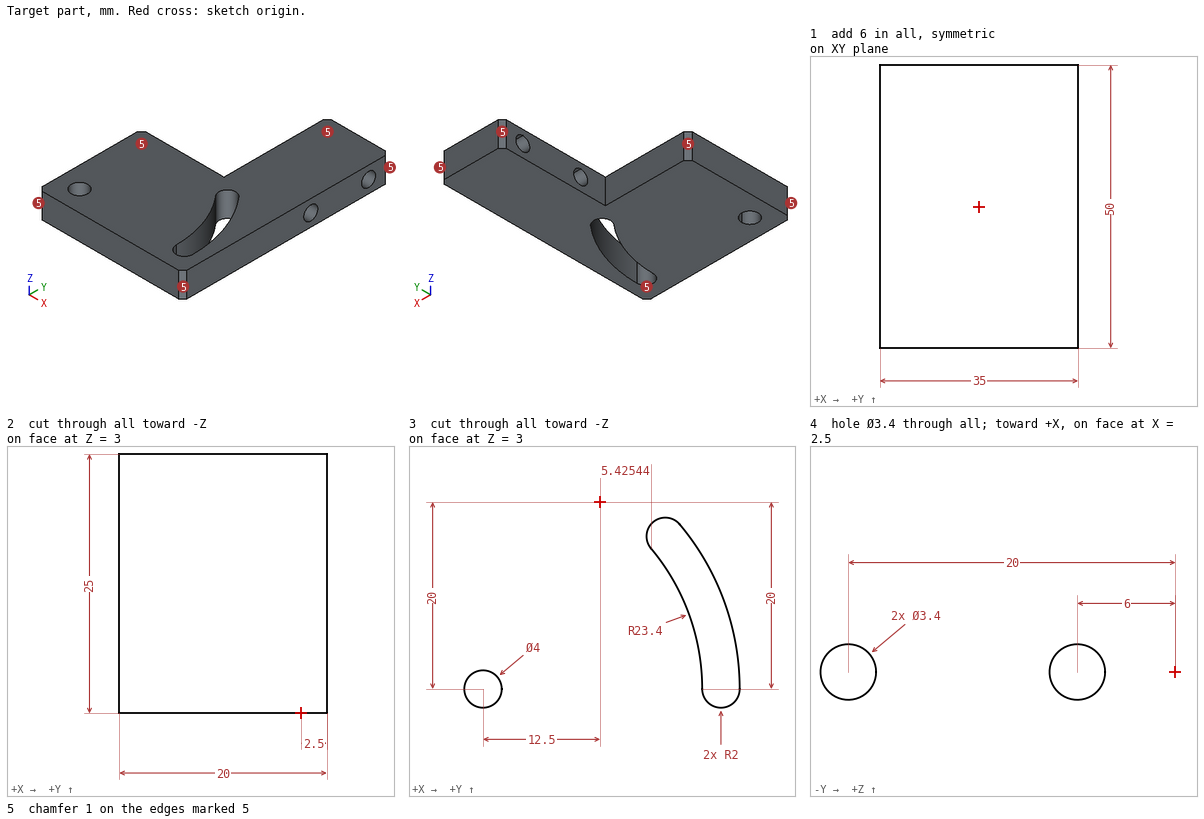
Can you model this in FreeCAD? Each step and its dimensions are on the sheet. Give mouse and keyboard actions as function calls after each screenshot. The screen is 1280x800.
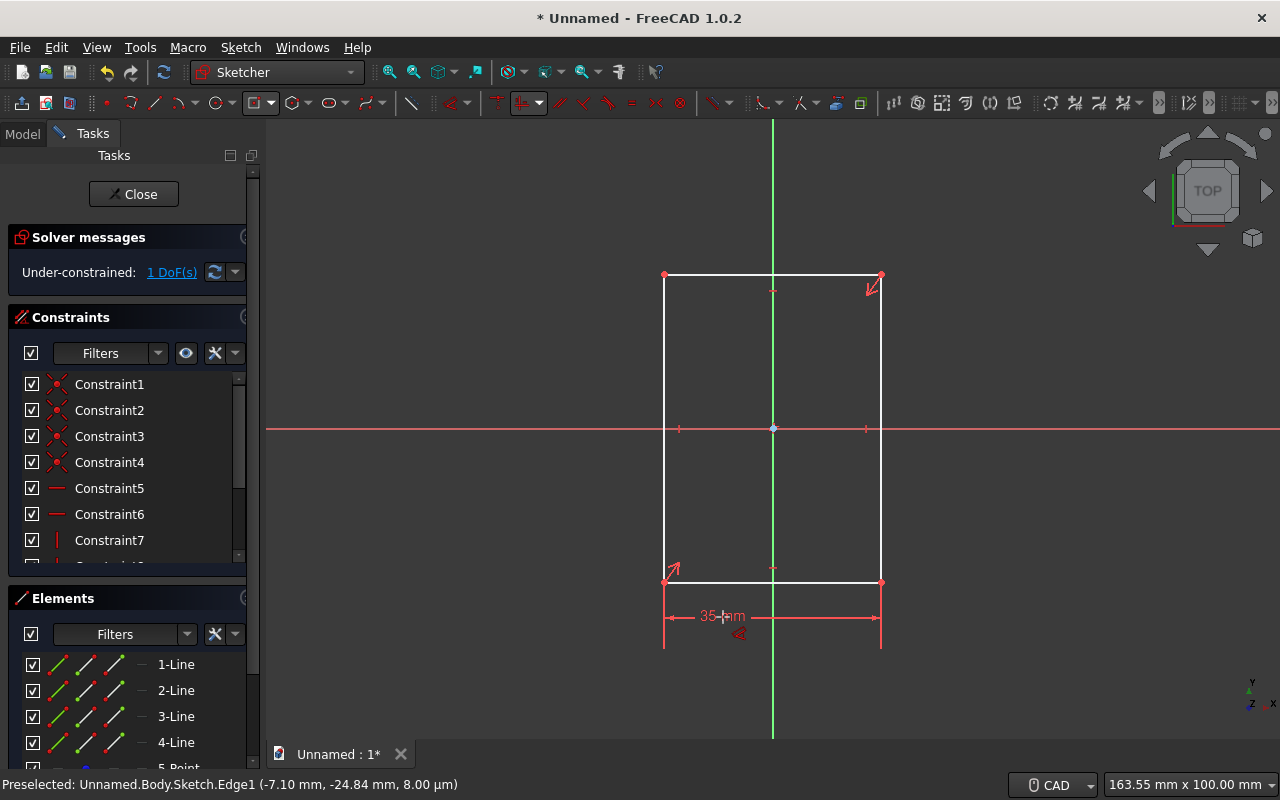
click(882, 491)
click(916, 358)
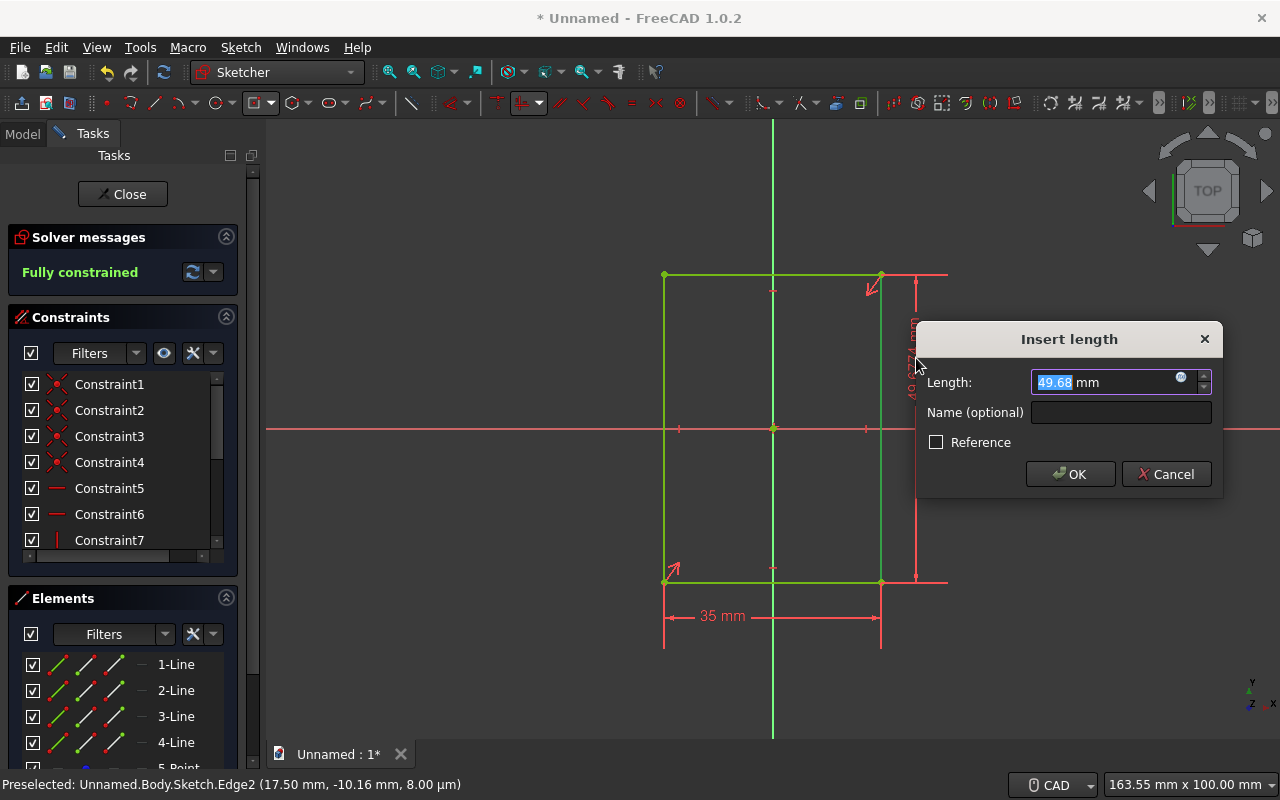
text(50)
key(Return)
key(Escape)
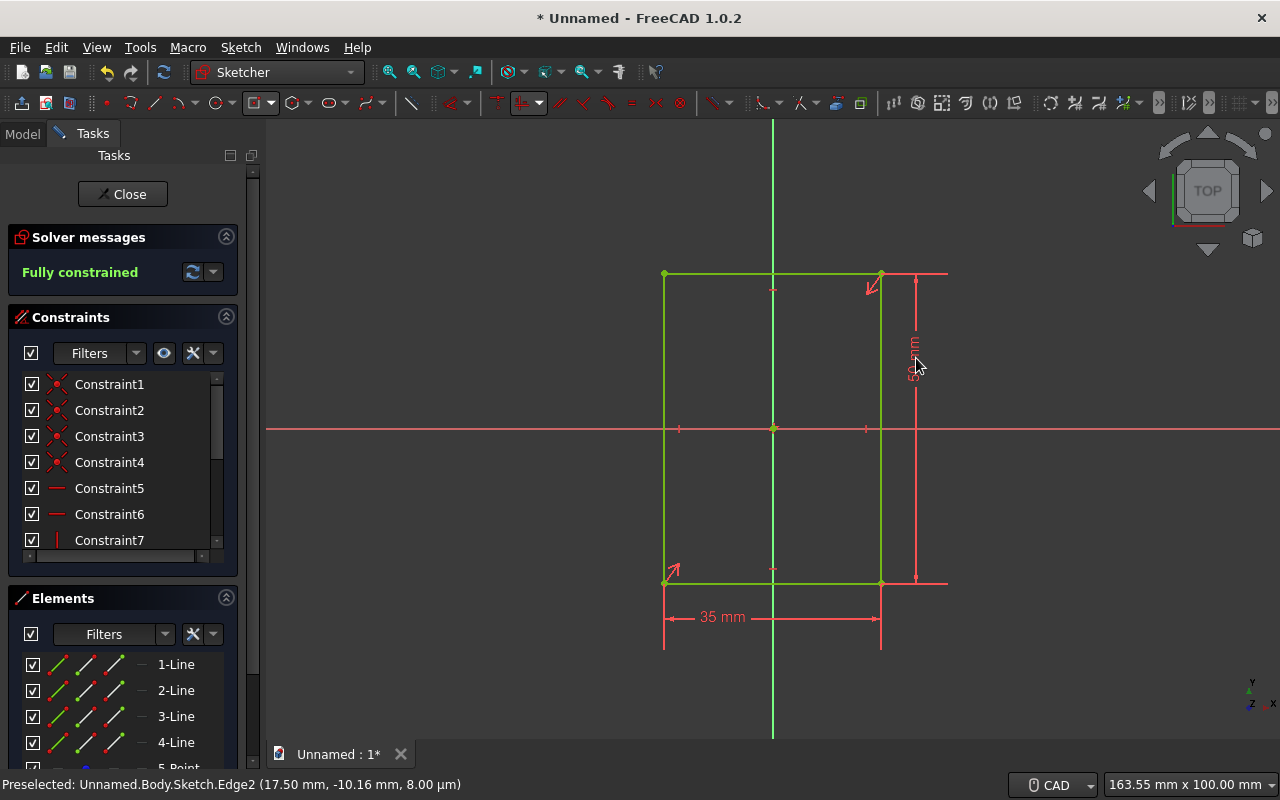
click(123, 194)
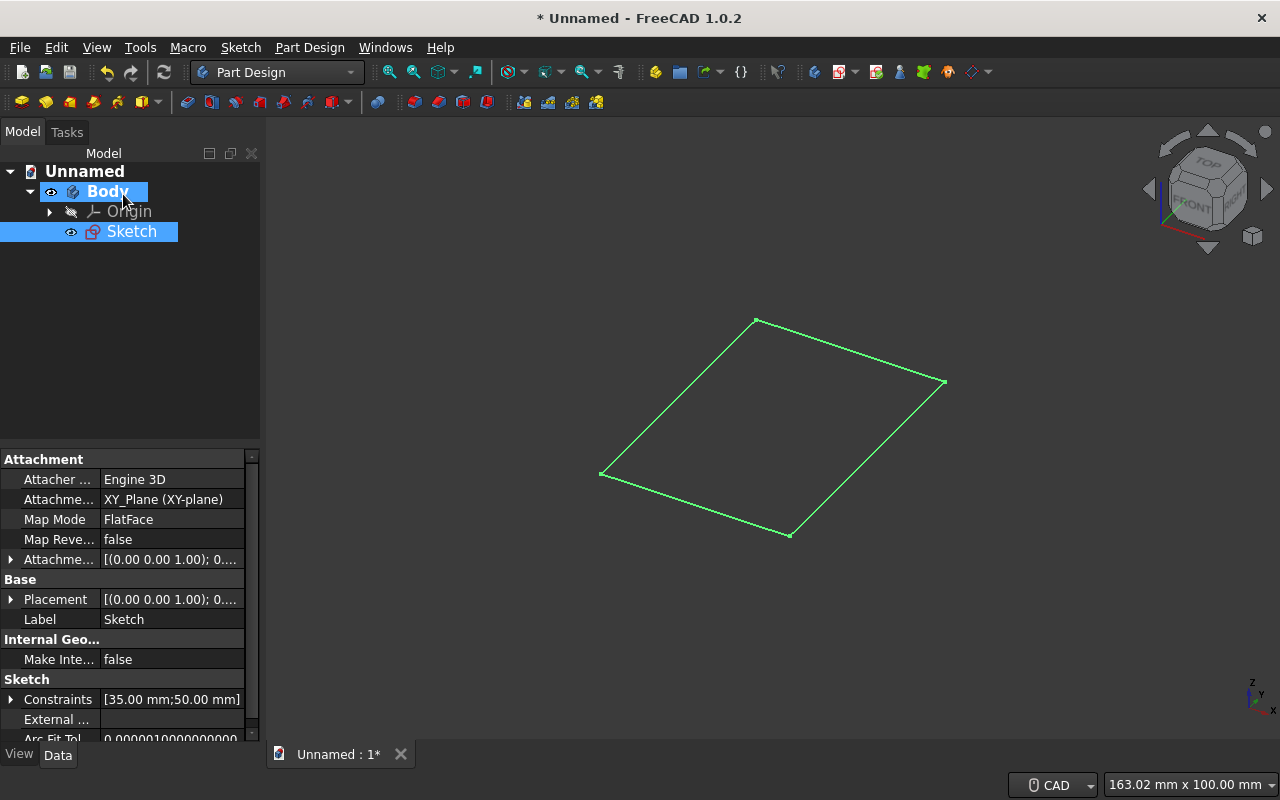
click(22, 102)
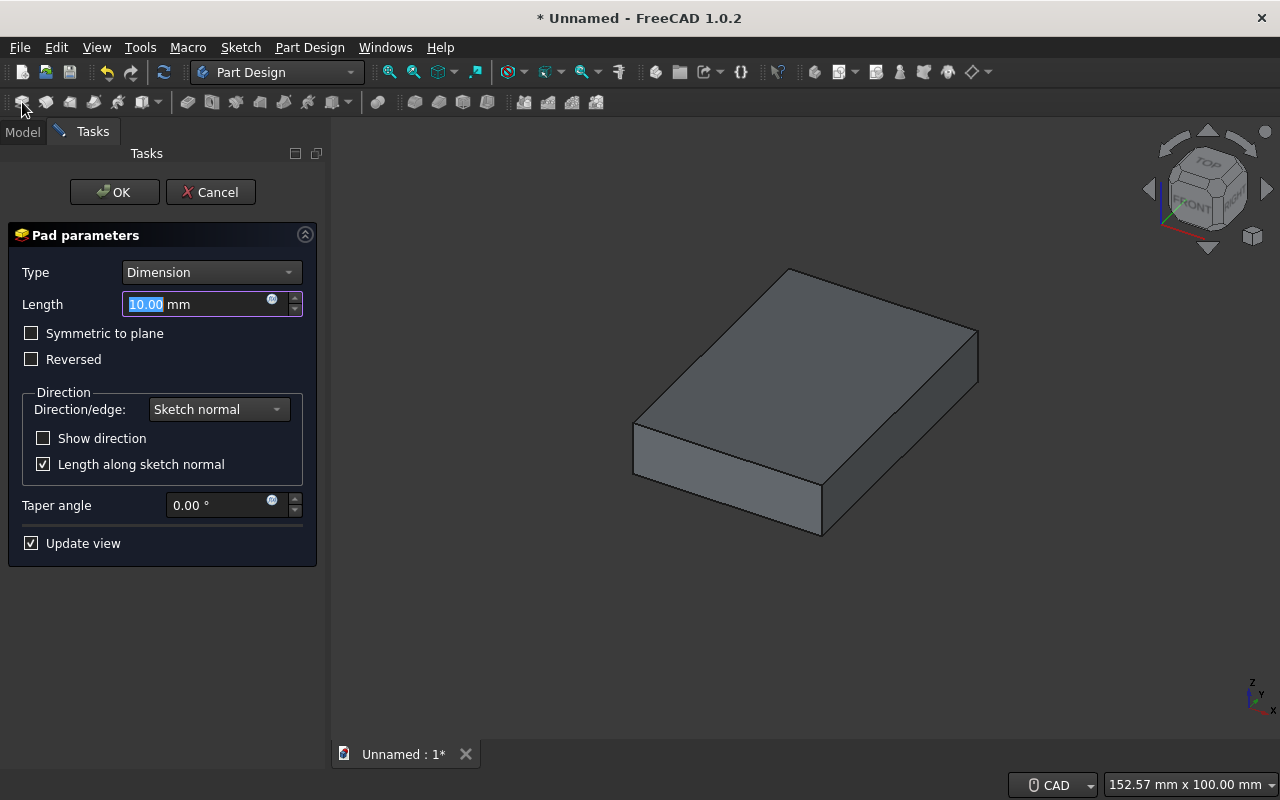
text(6)
key(Tab)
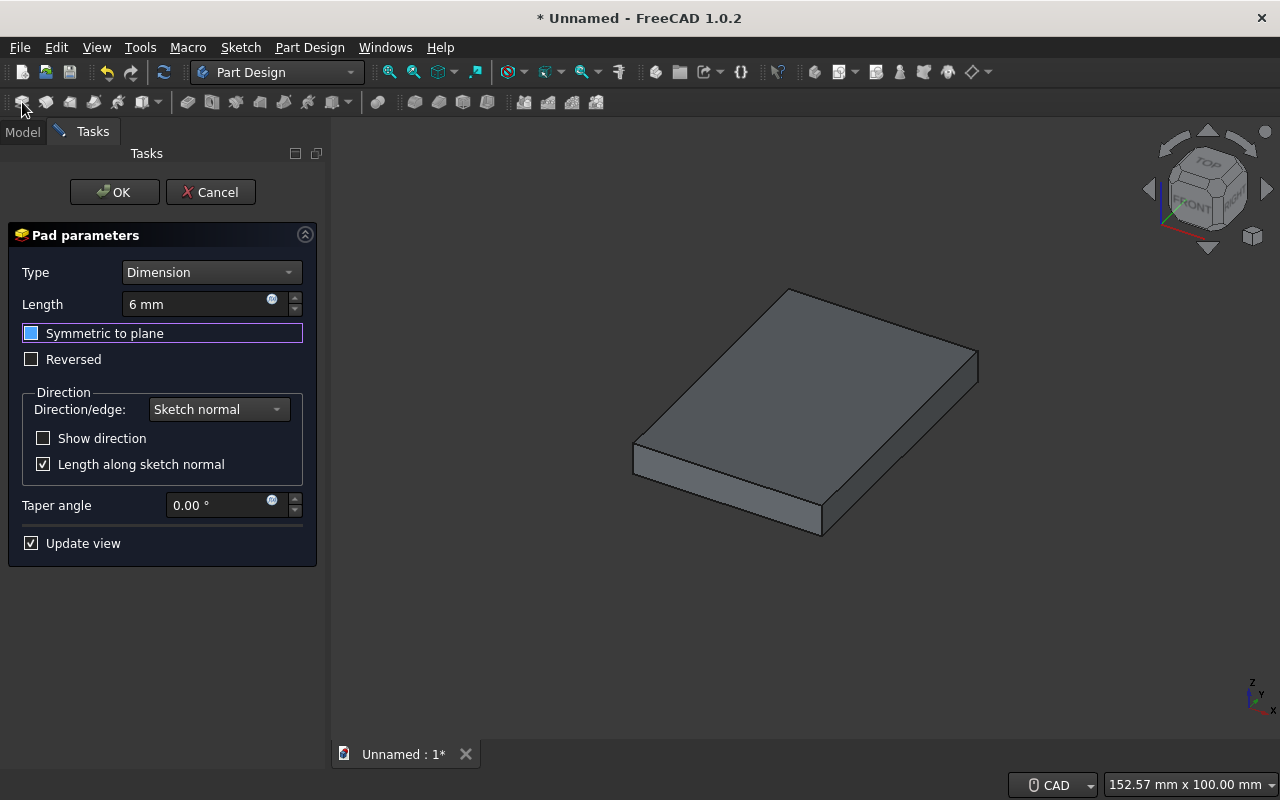
click(30, 333)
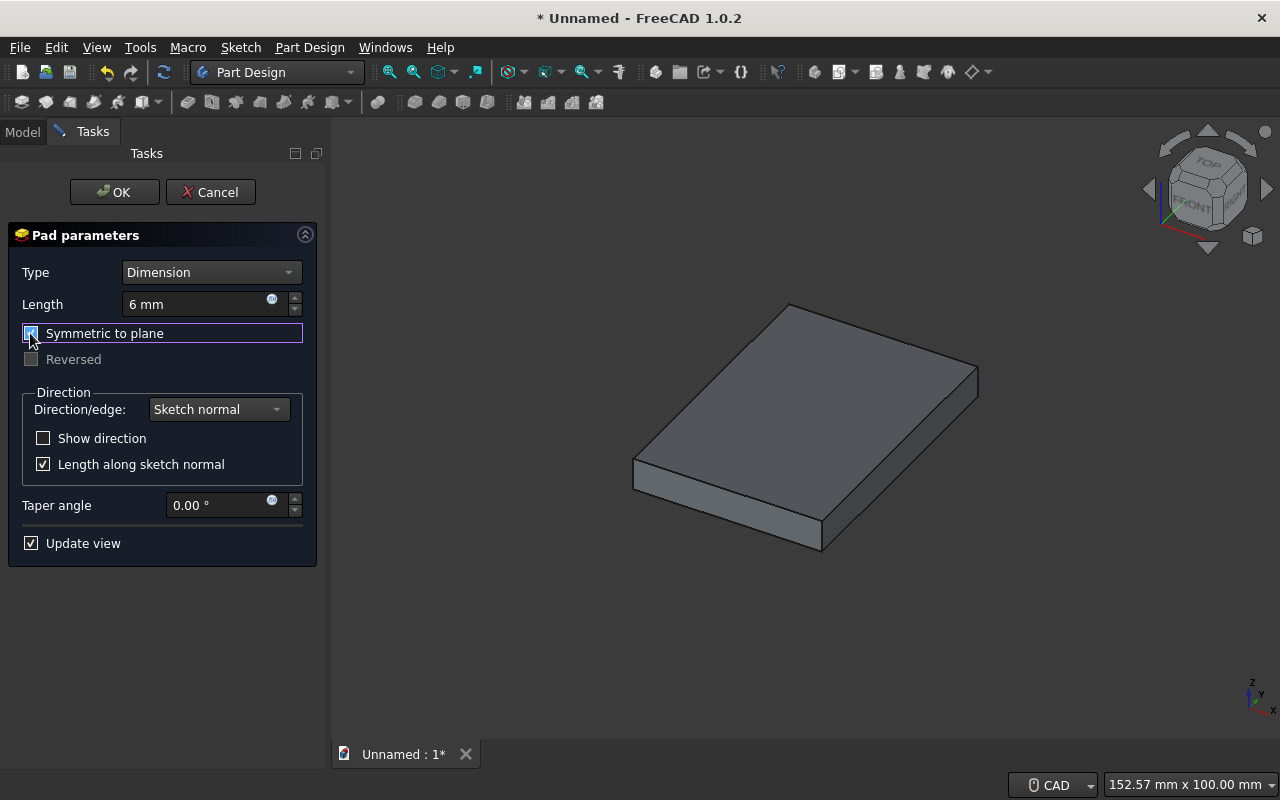
click(115, 192)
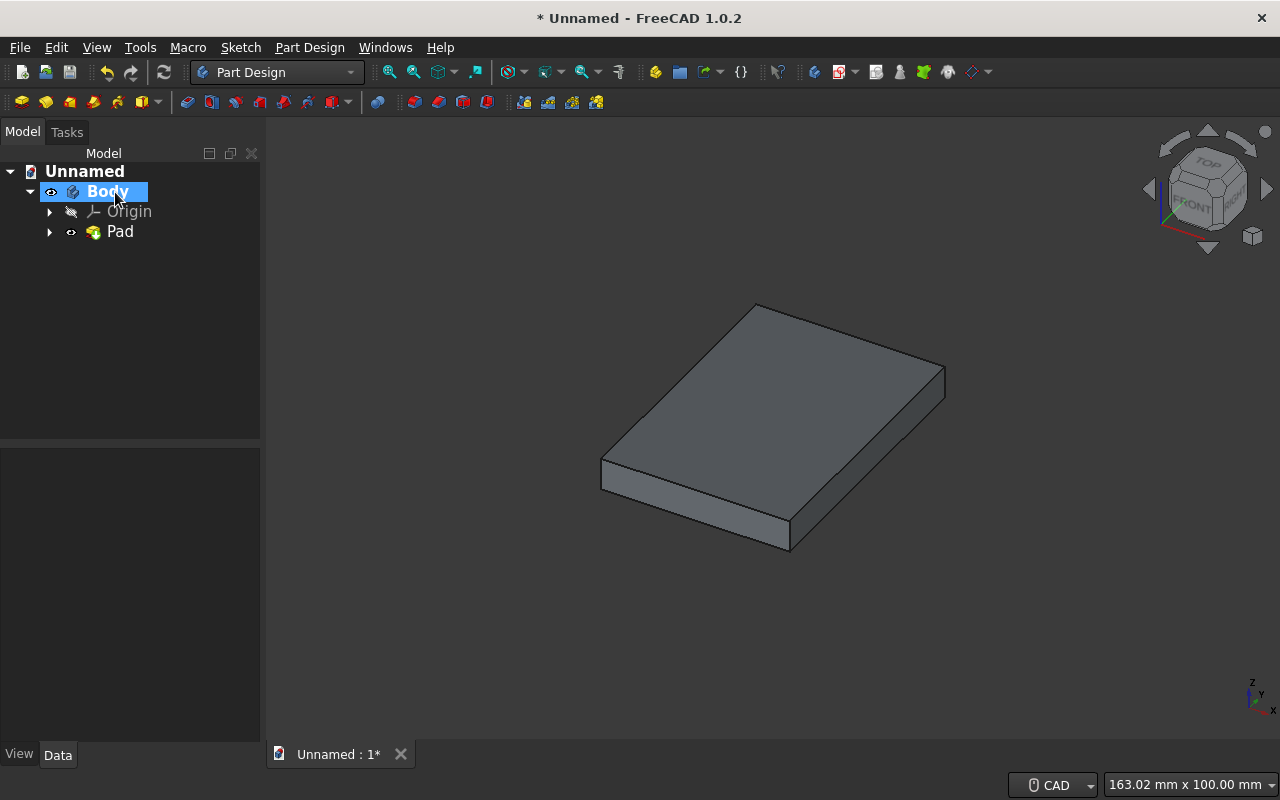
click(390, 72)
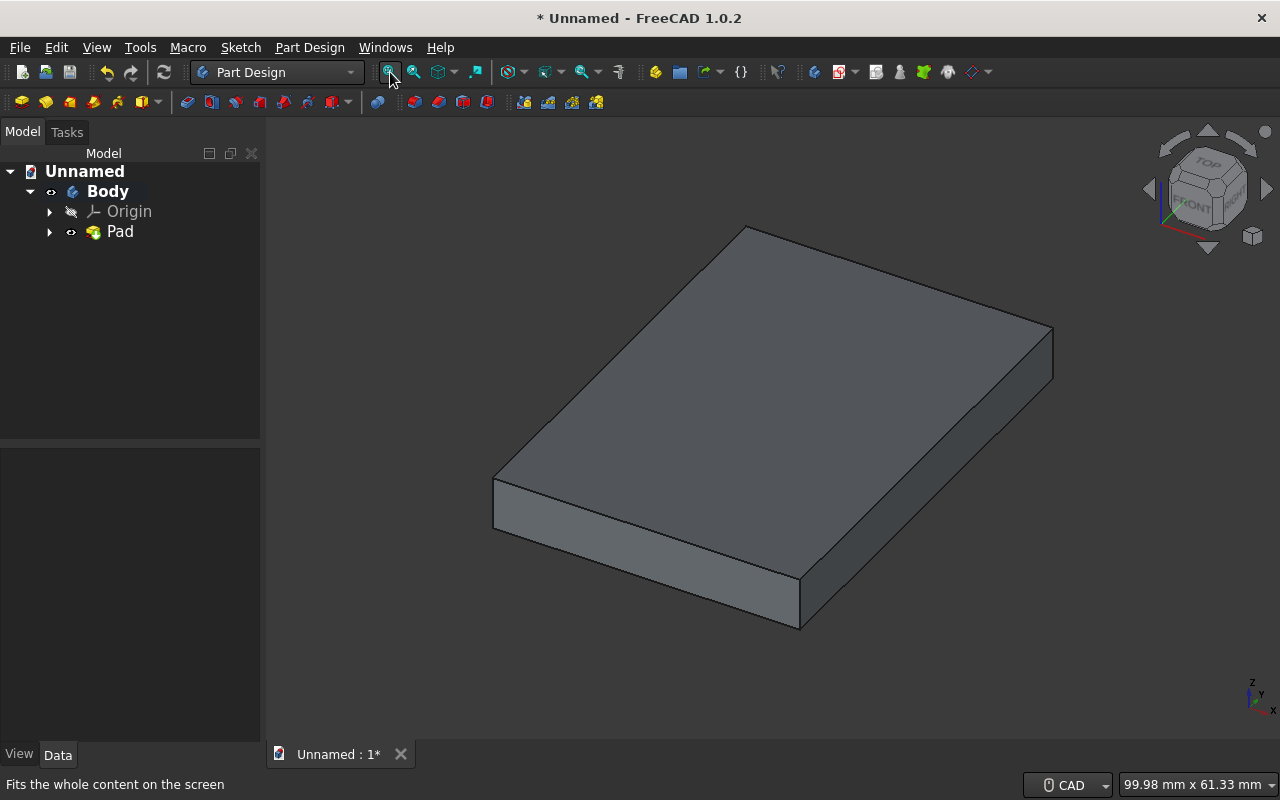
click(809, 366)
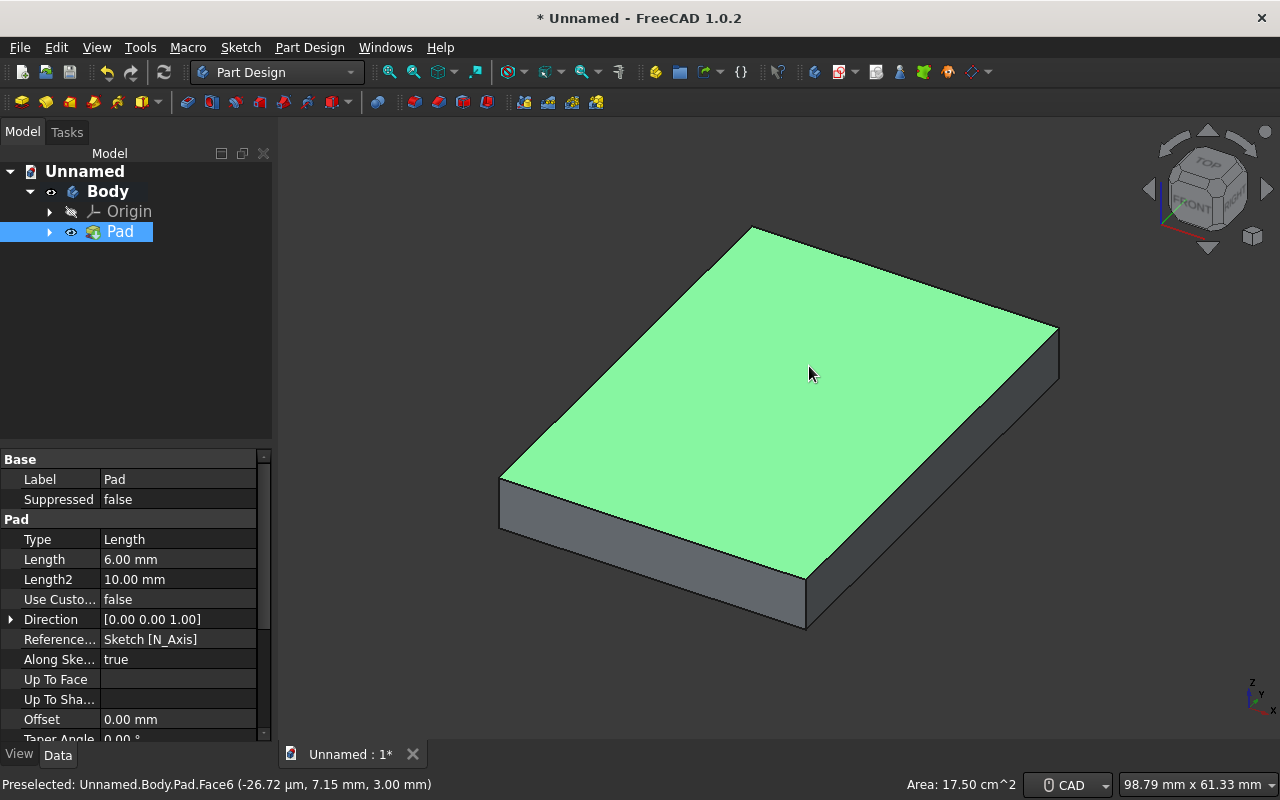
click(840, 72)